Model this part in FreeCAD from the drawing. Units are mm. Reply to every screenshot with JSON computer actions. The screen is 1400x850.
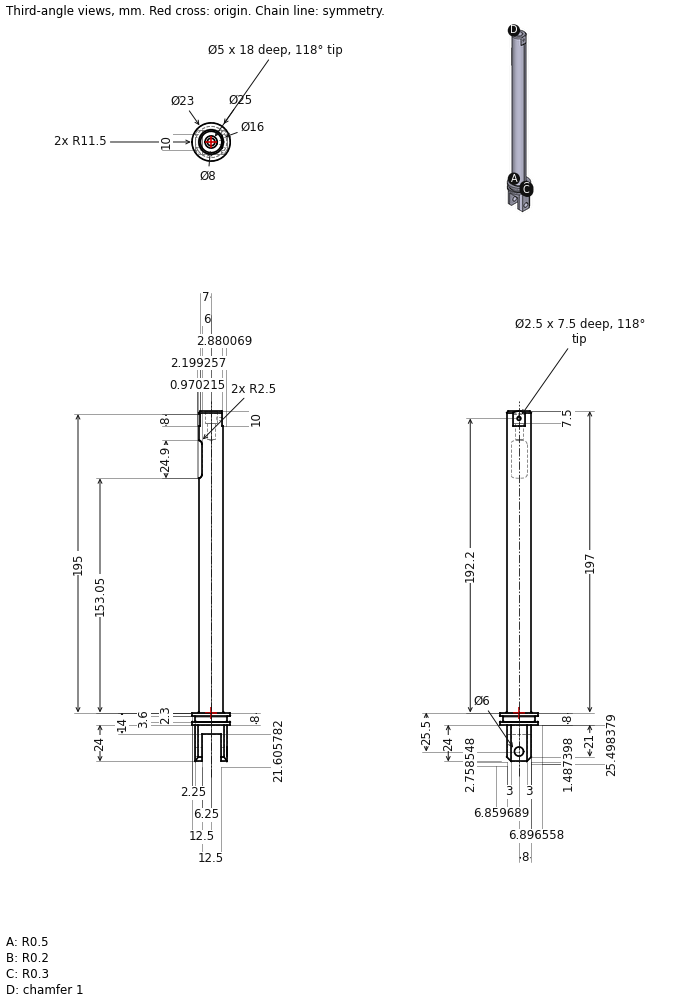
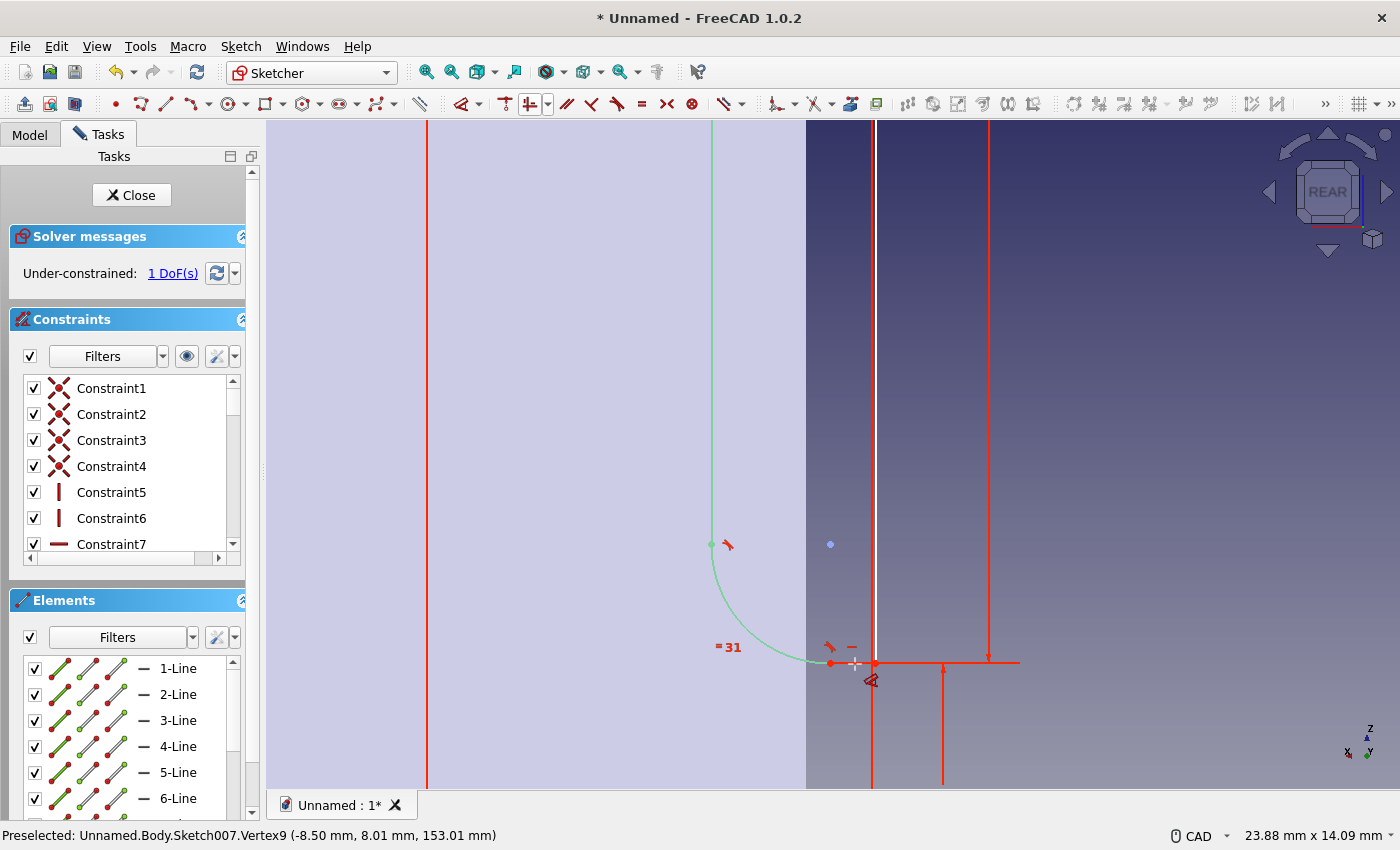
{"action": "left_click", "coordinate": [853, 663]}
{"action": "left_click", "coordinate": [853, 697]}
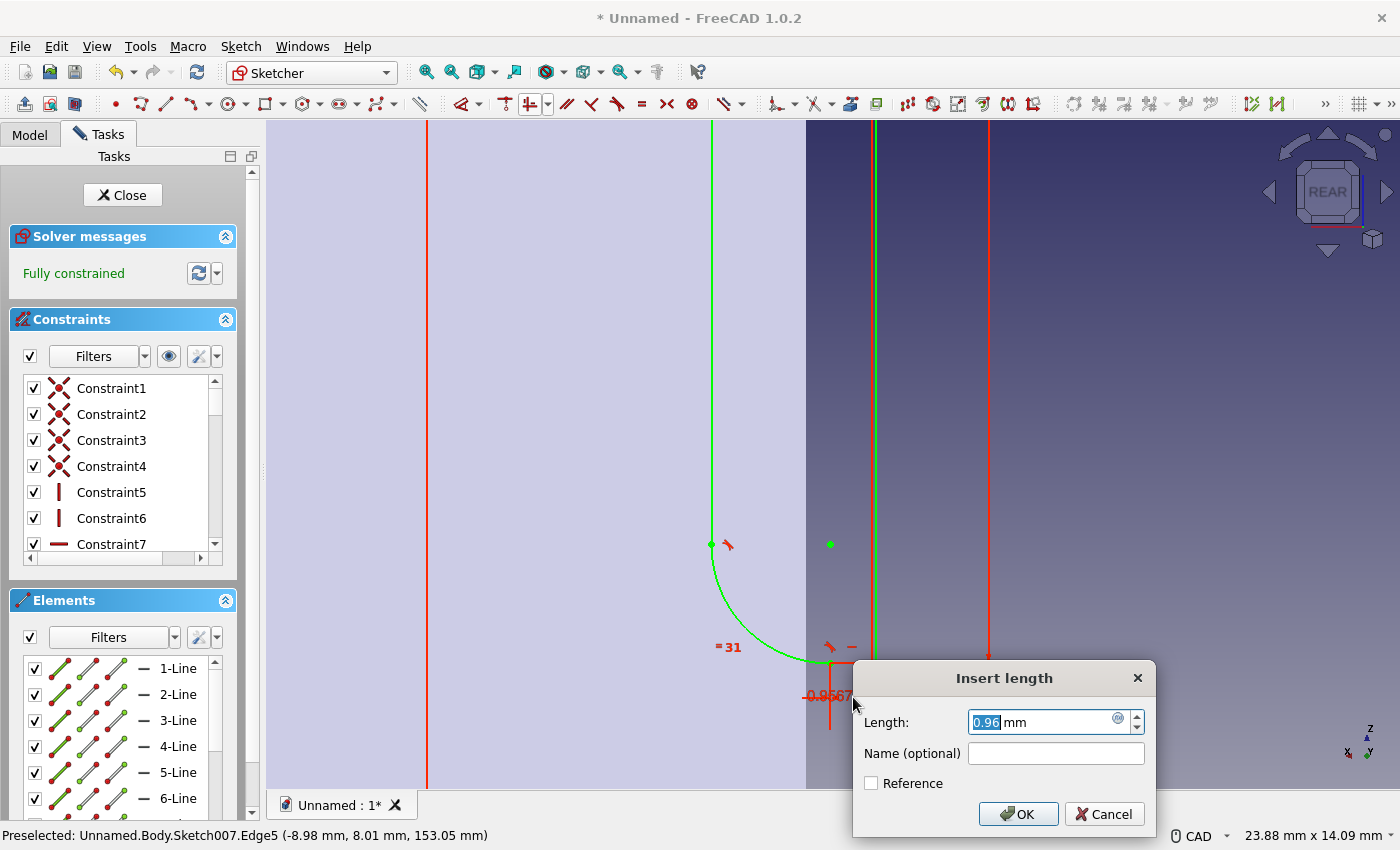
{"action": "type", "text": "0.970215"}
{"action": "key", "text": "Return"}
{"action": "key", "text": "Escape"}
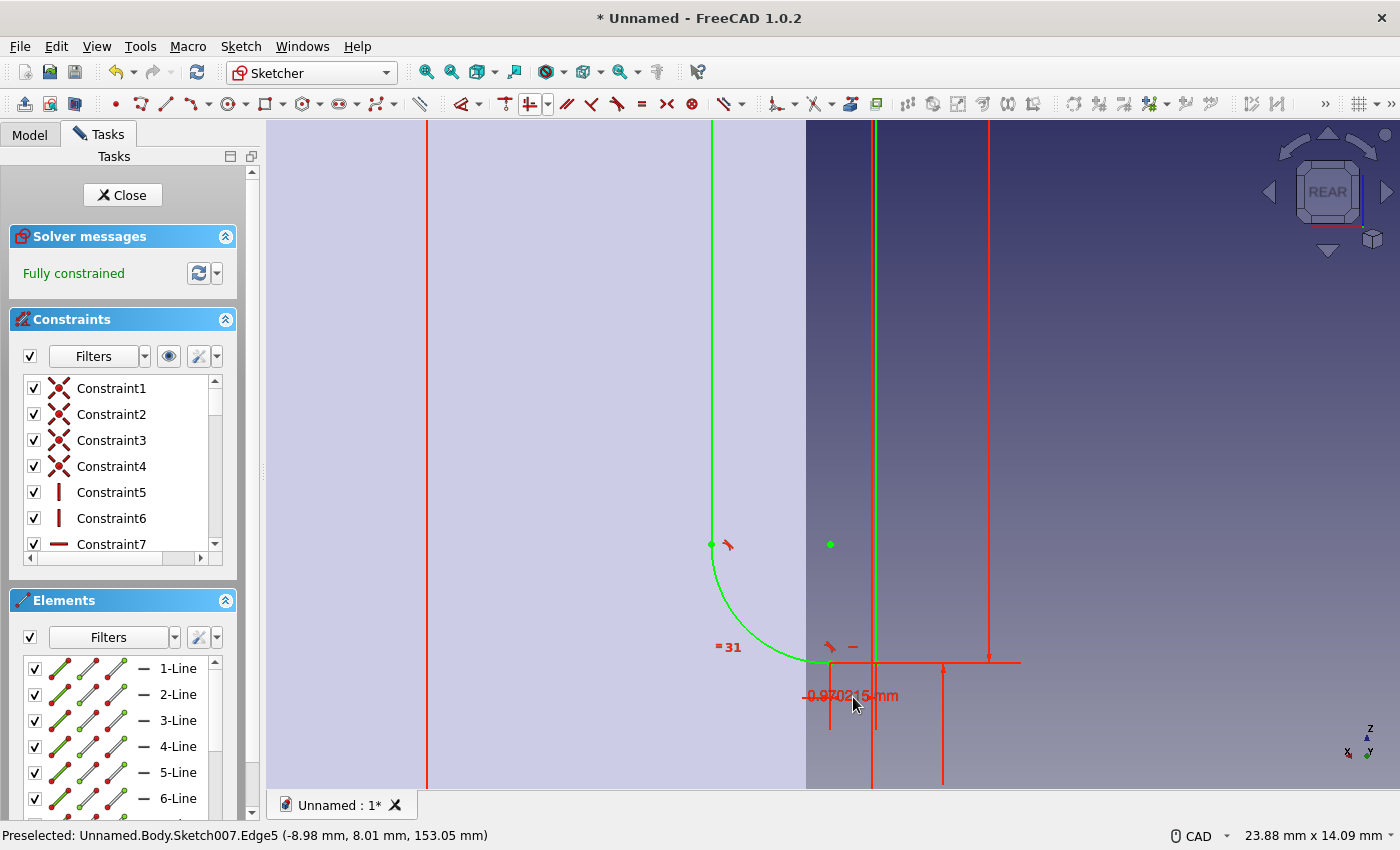
{"action": "left_click", "coordinate": [123, 195]}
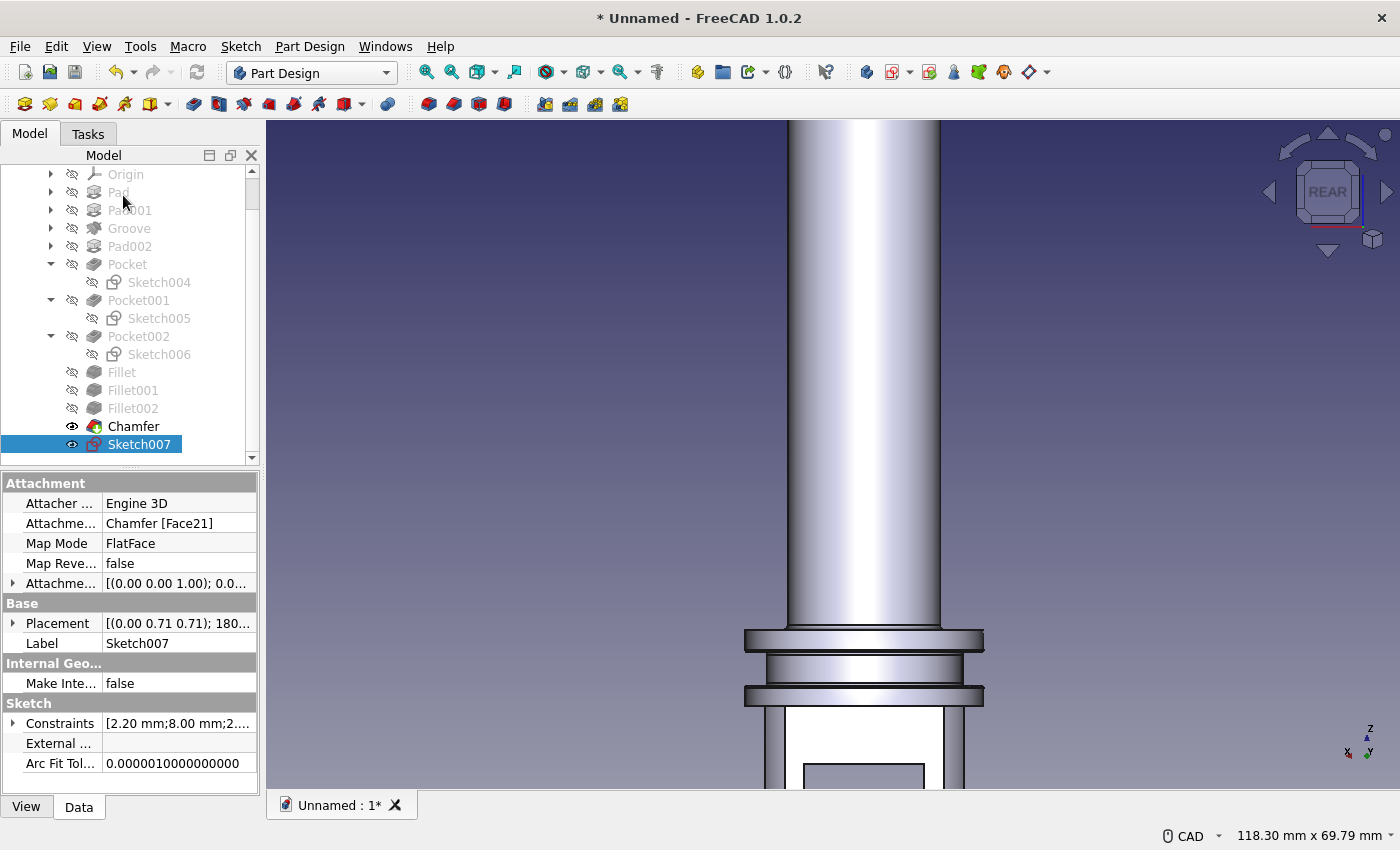
{"action": "left_click", "coordinate": [194, 104]}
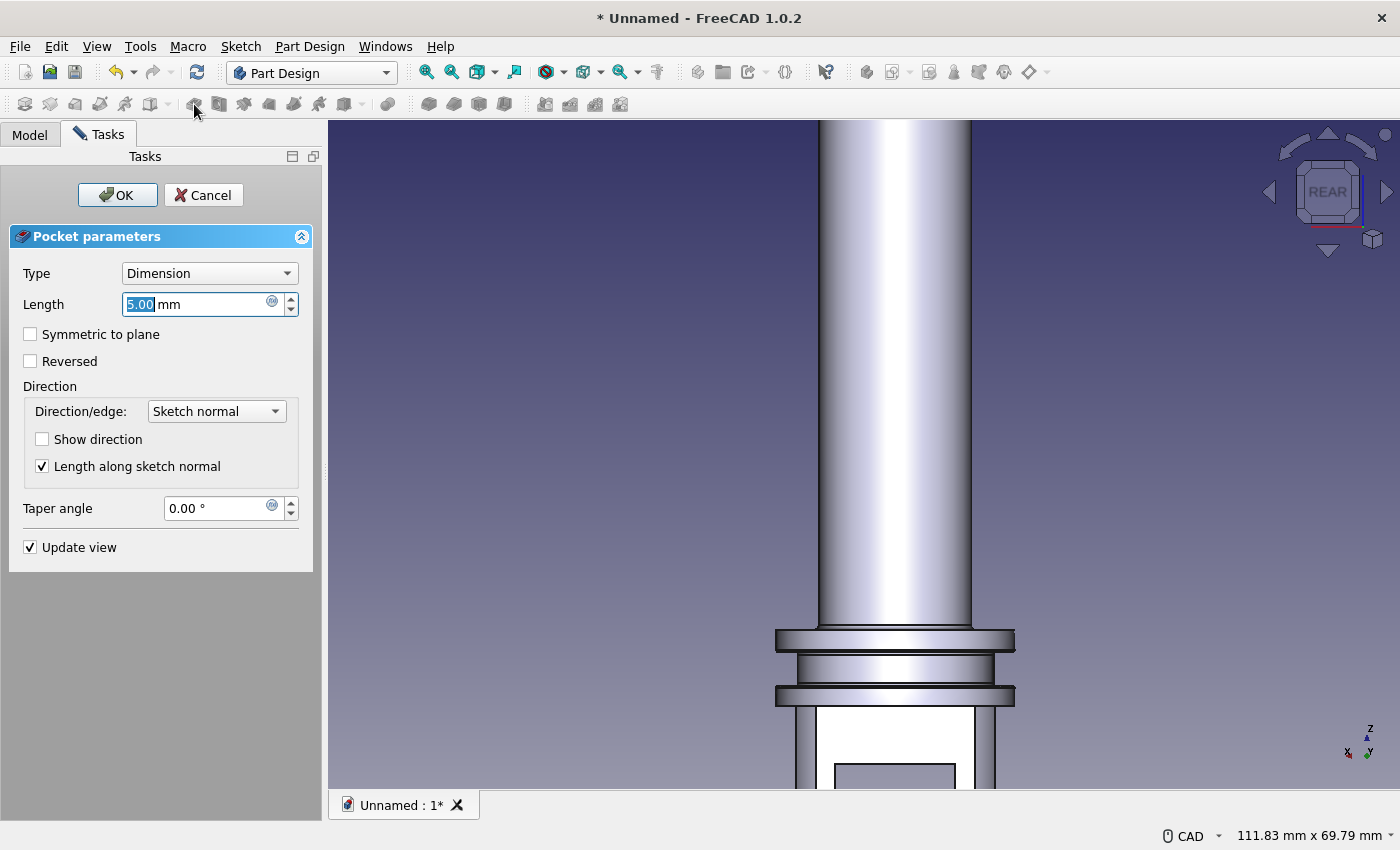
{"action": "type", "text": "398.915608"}
{"action": "key", "text": "Tab"}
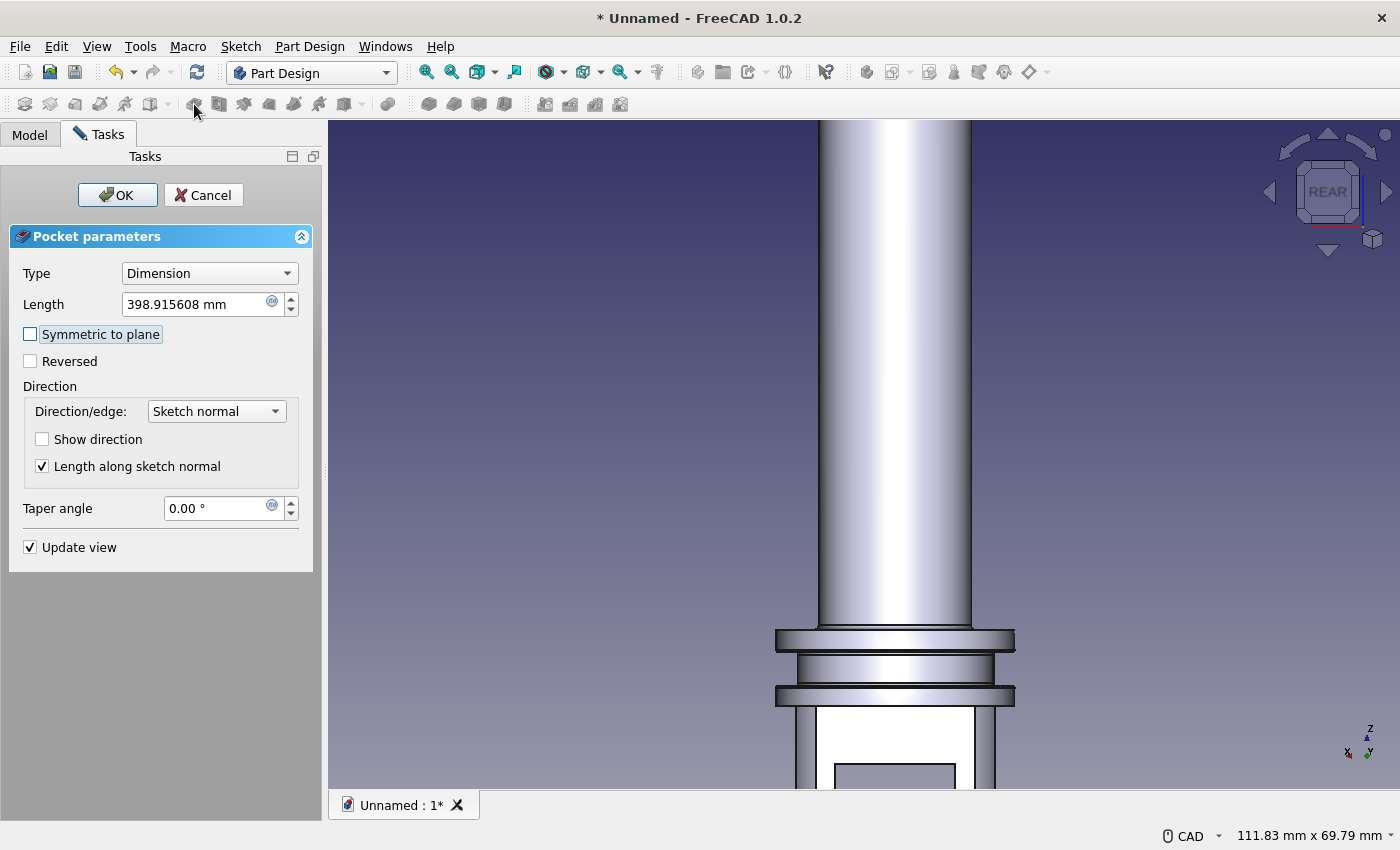
{"action": "left_click", "coordinate": [31, 334]}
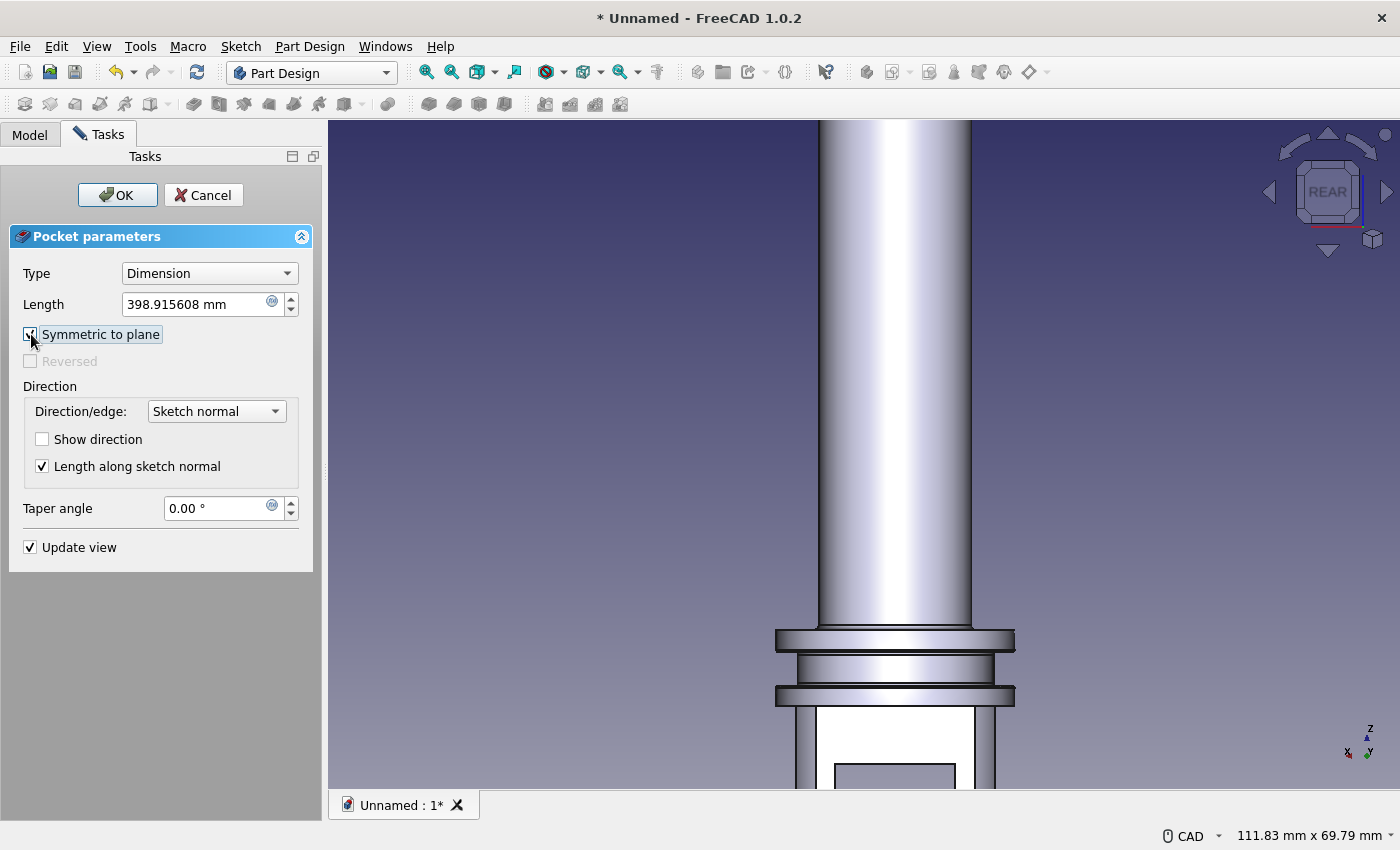
{"action": "left_click", "coordinate": [118, 195]}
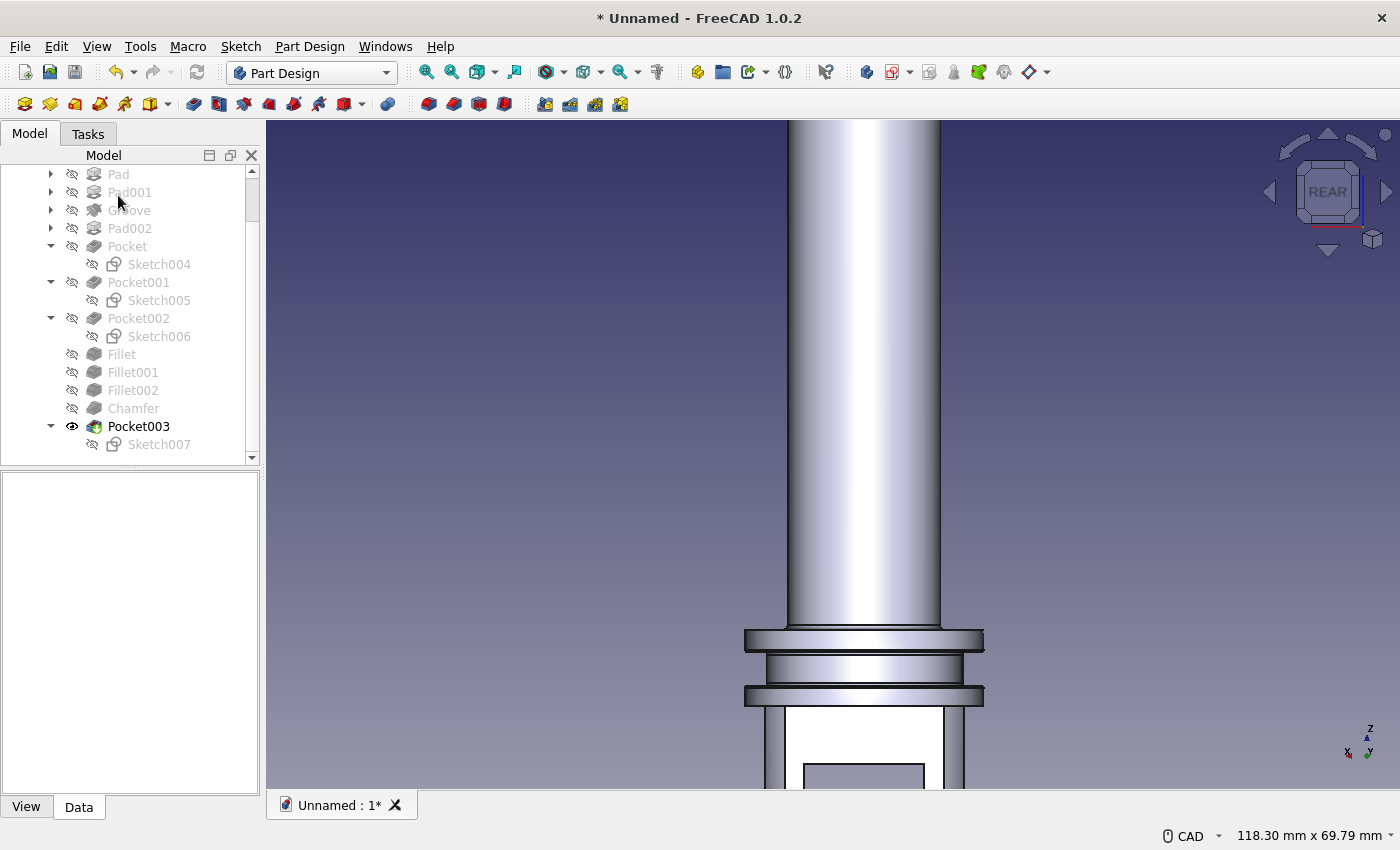
{"action": "left_click", "coordinate": [427, 72]}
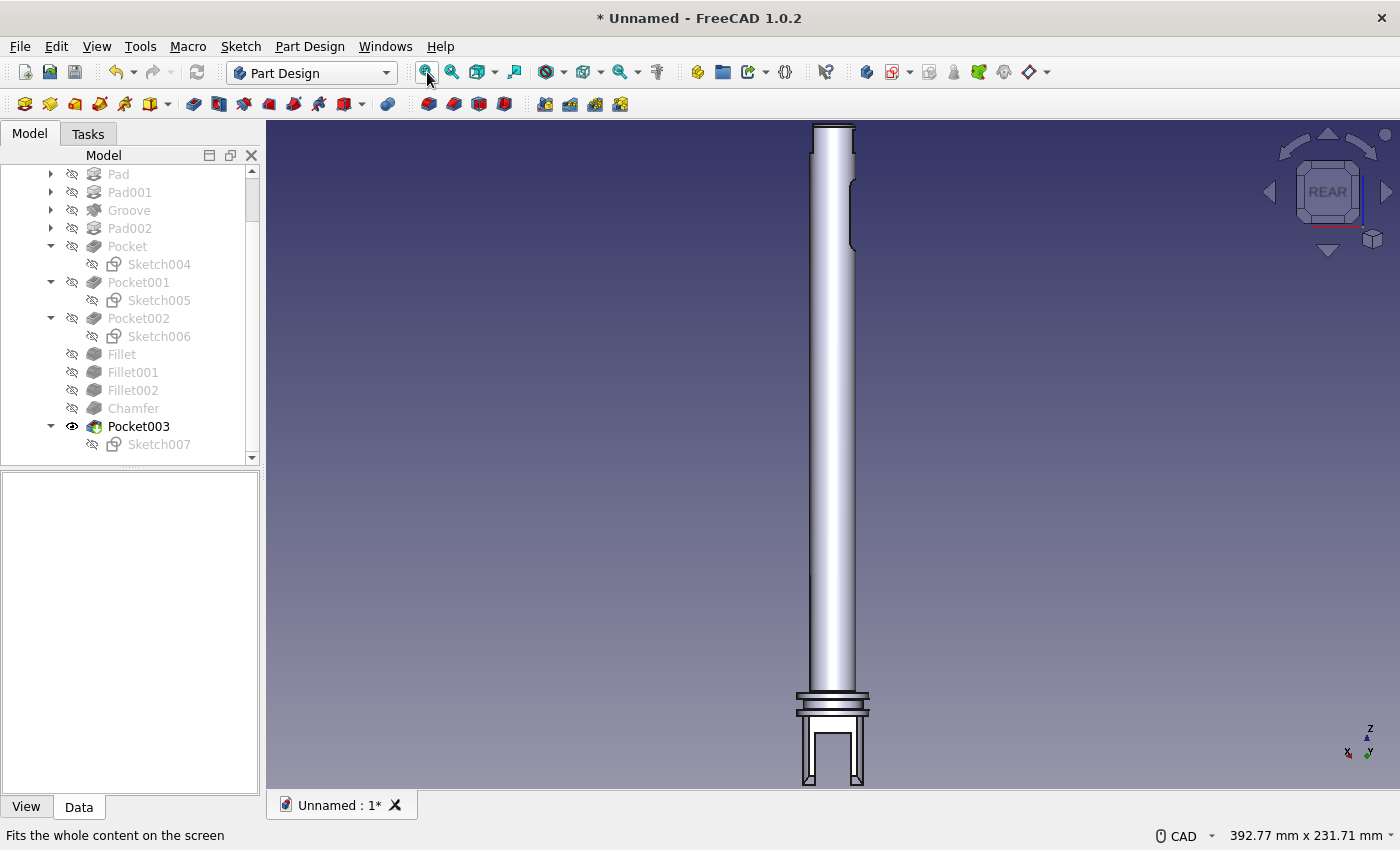
{"action": "key", "text": "0"}